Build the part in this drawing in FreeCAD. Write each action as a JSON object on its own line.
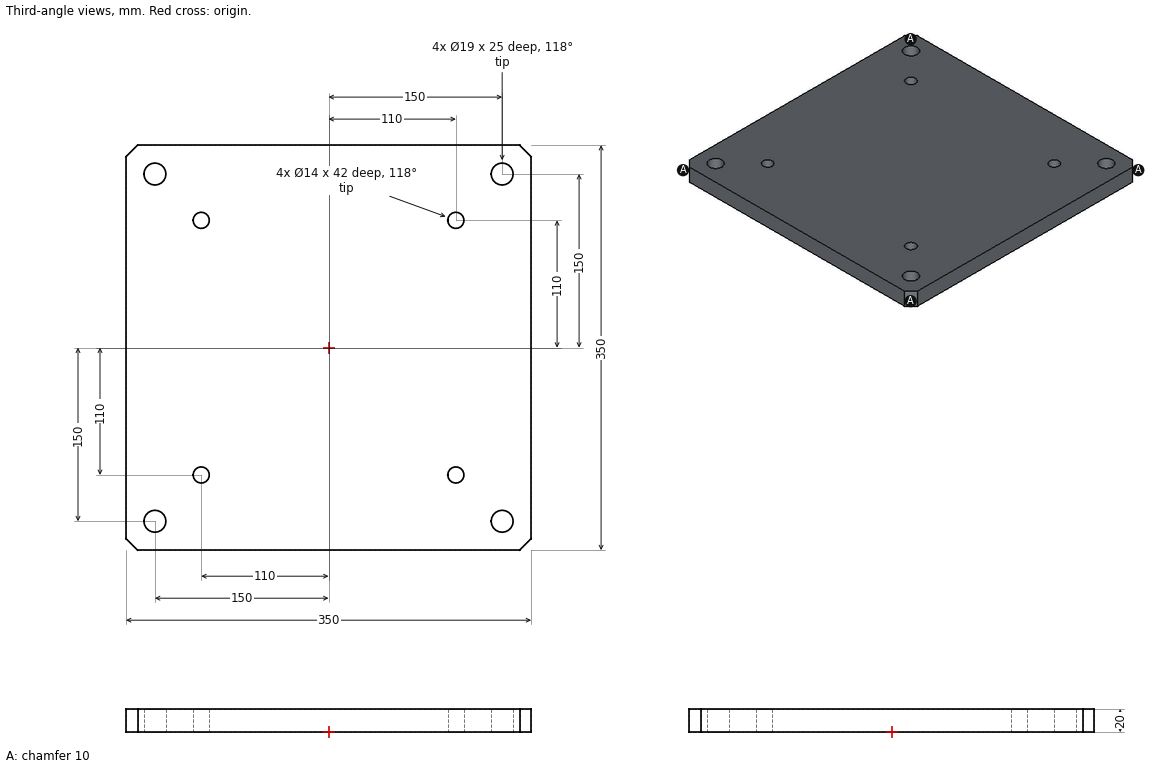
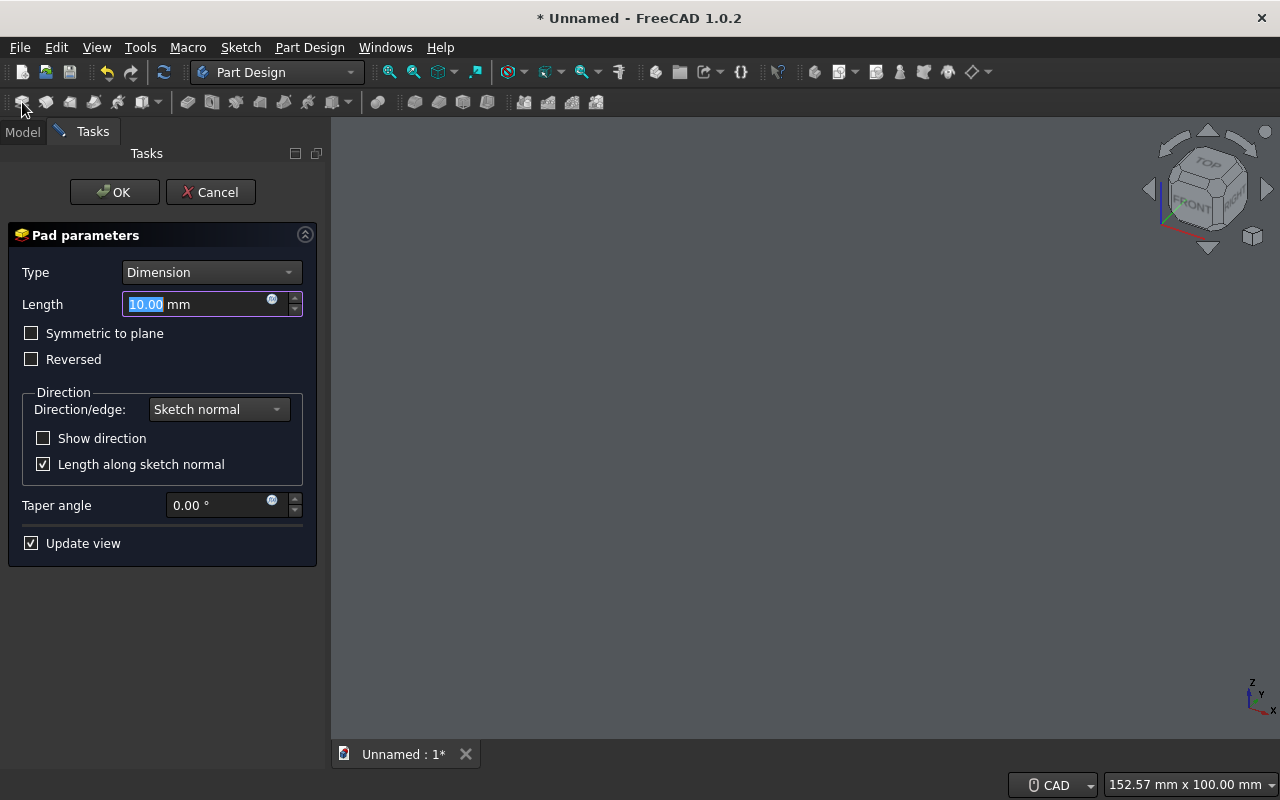
{"action": "type", "text": "20"}
{"action": "key", "text": "Tab"}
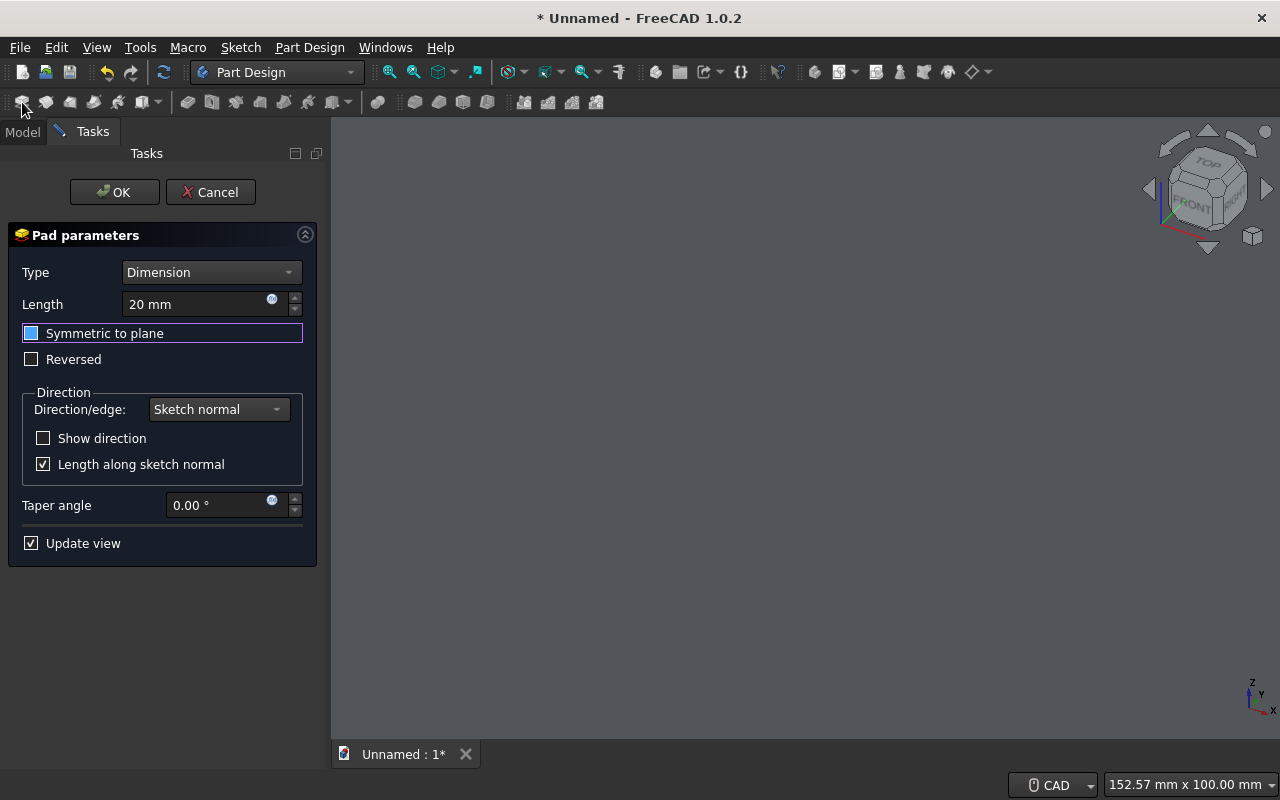
{"action": "left_click", "coordinate": [115, 192]}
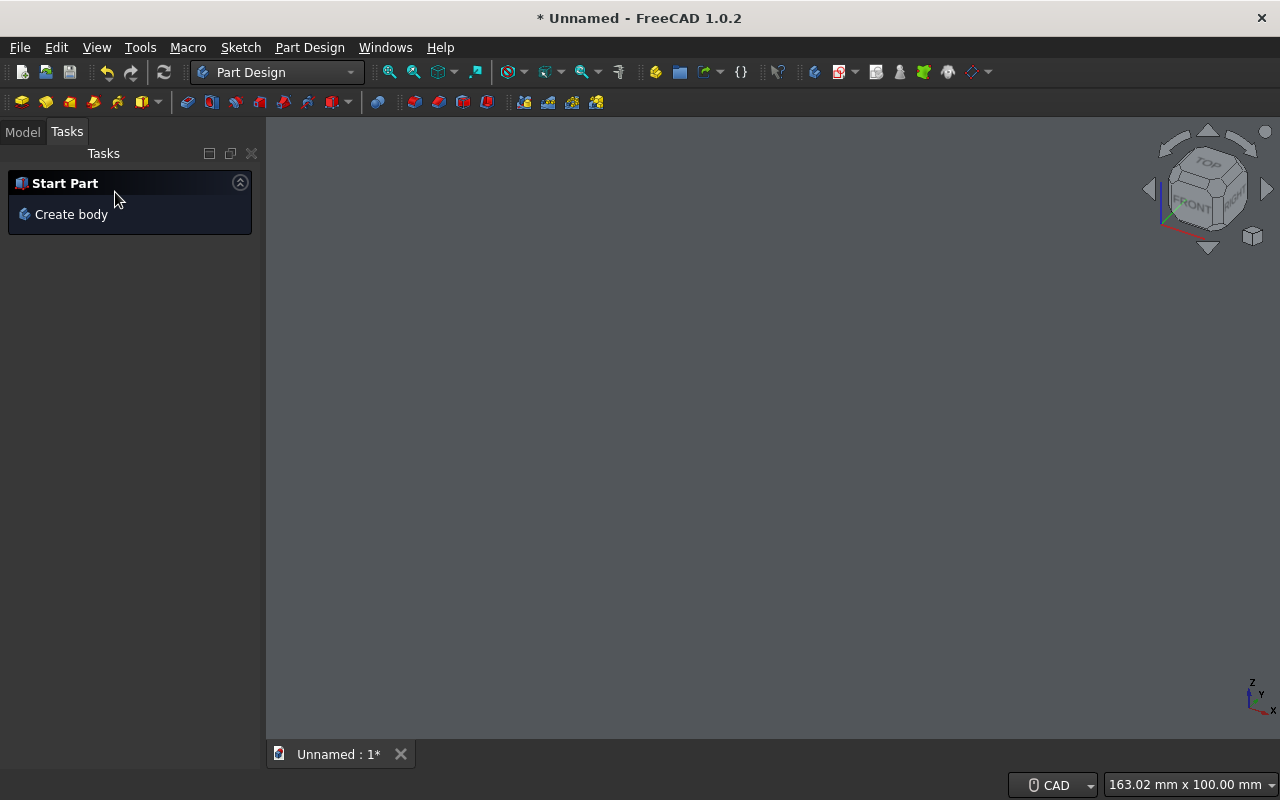
{"action": "left_click", "coordinate": [390, 72]}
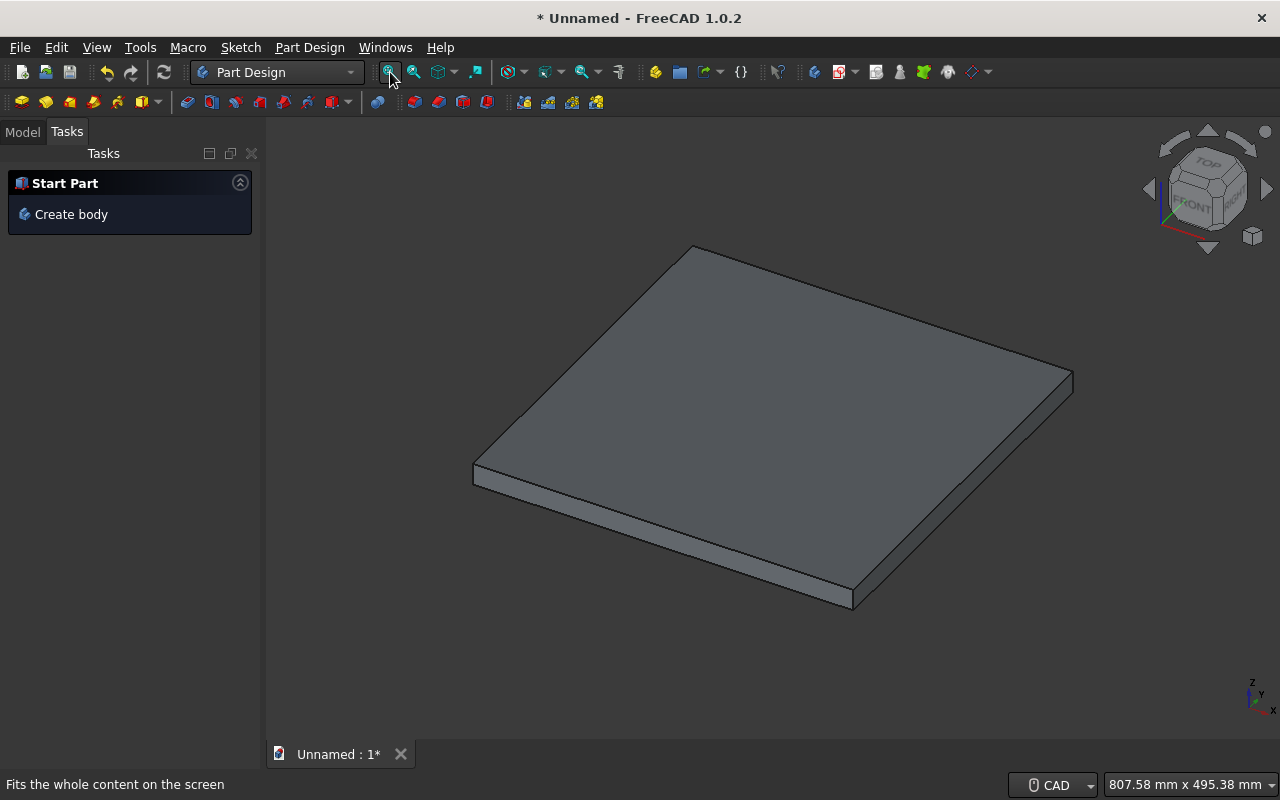
{"action": "left_click", "coordinate": [773, 417]}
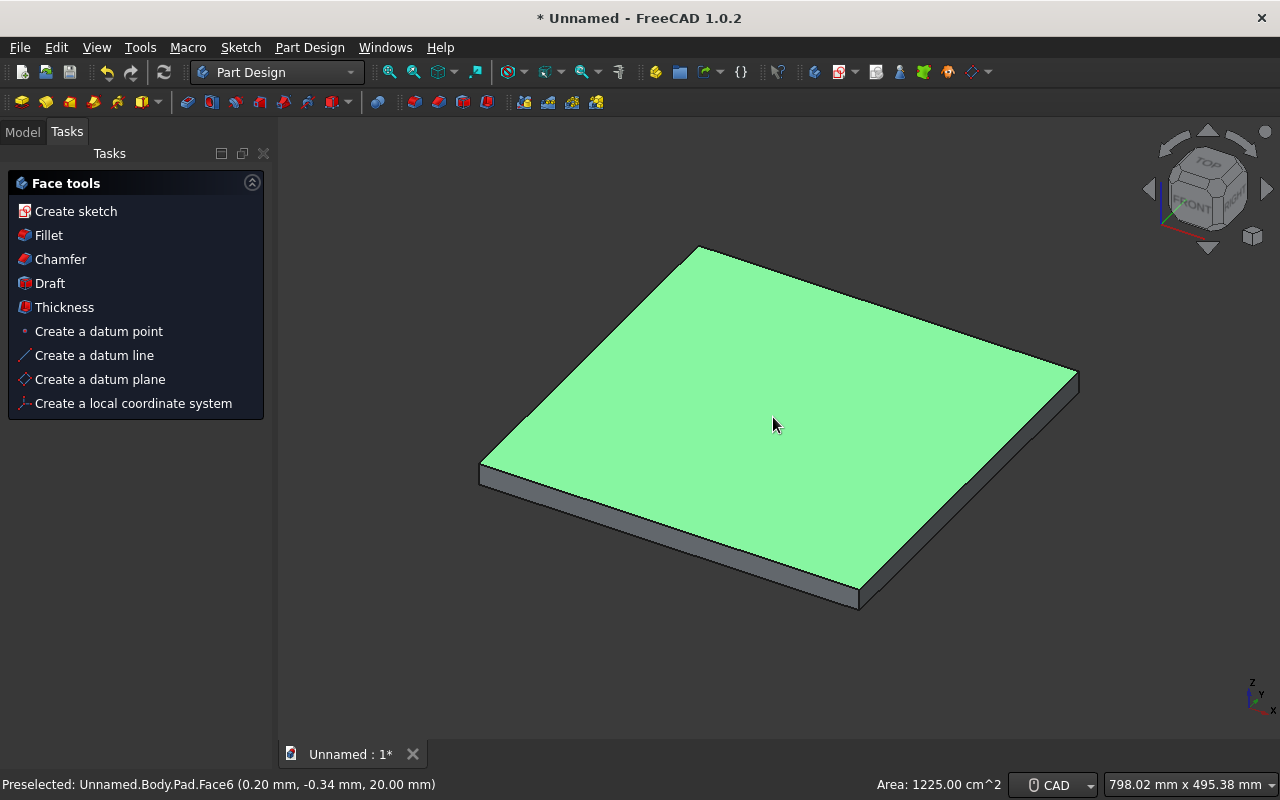
{"action": "left_click", "coordinate": [840, 72]}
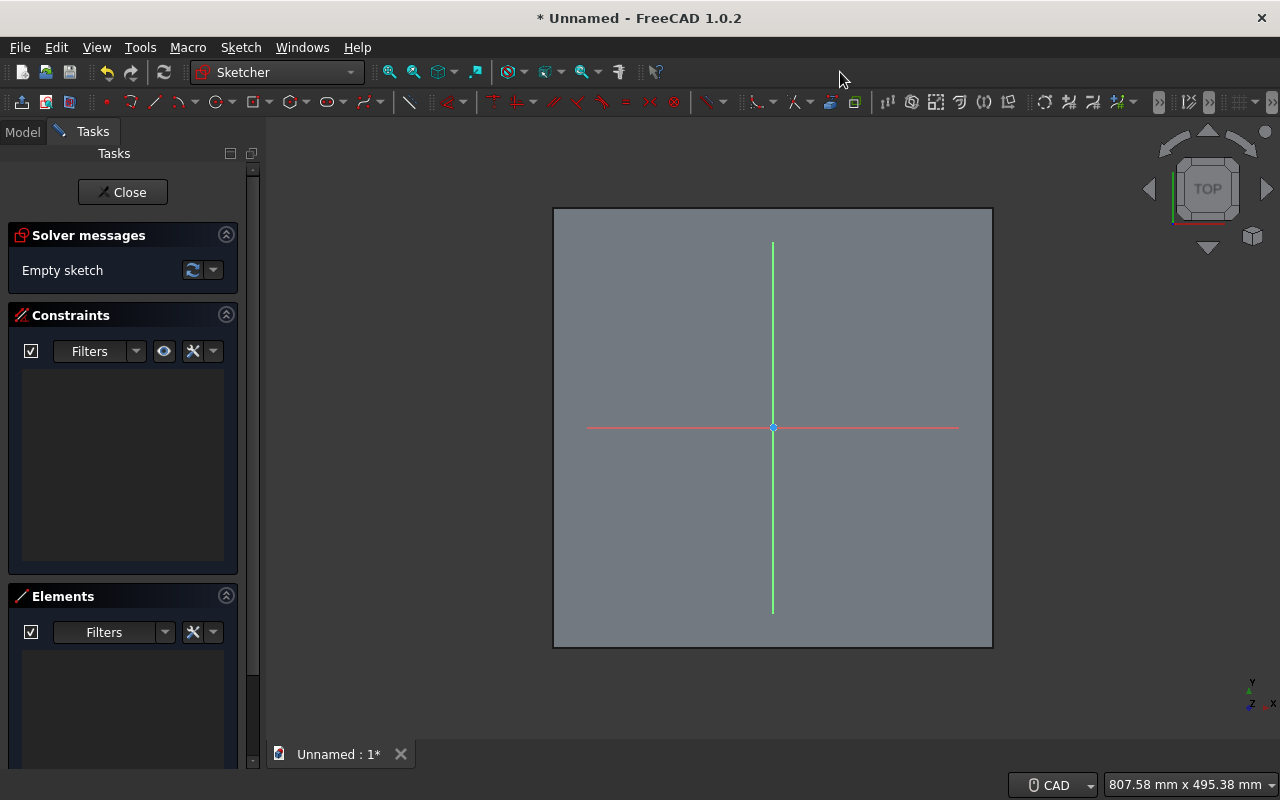
{"action": "scroll", "coordinate": [912, 428], "scroll_direction": "up", "scroll_amount": 2}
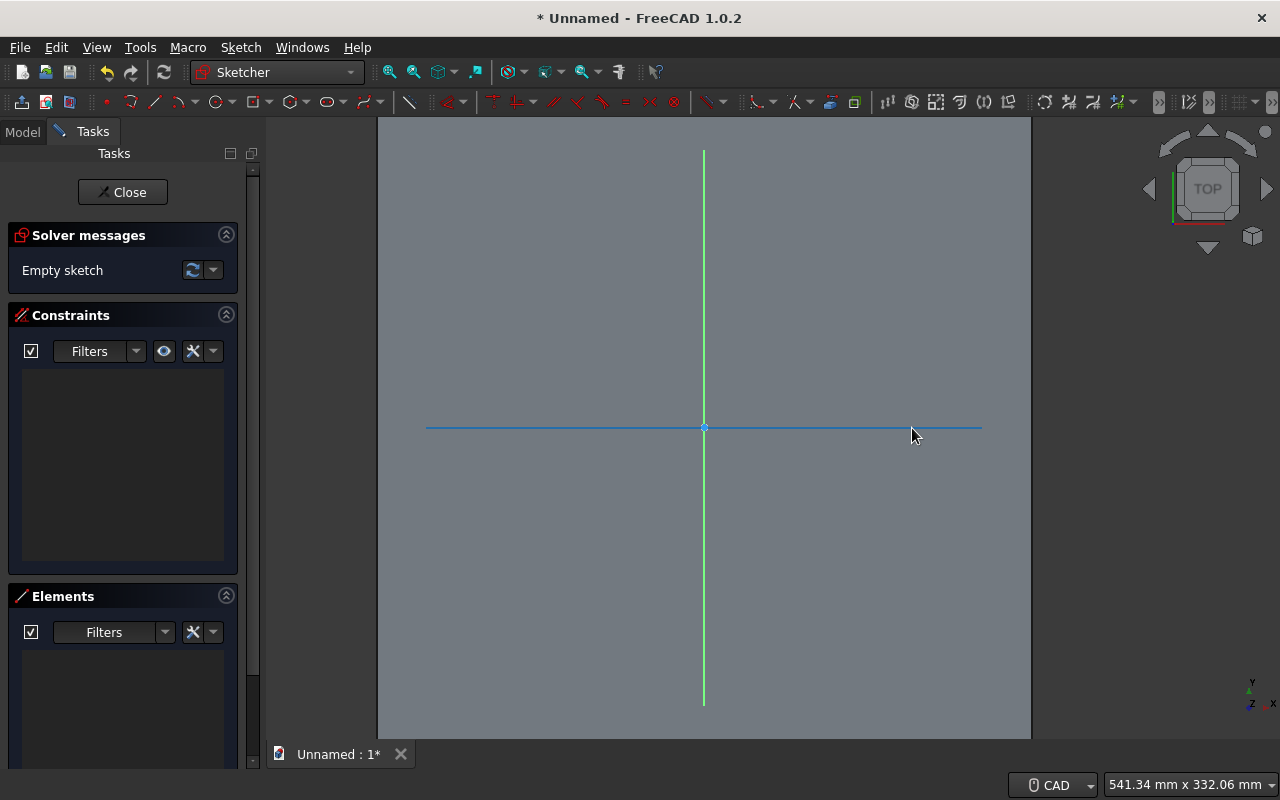
{"action": "key", "text": "g c"}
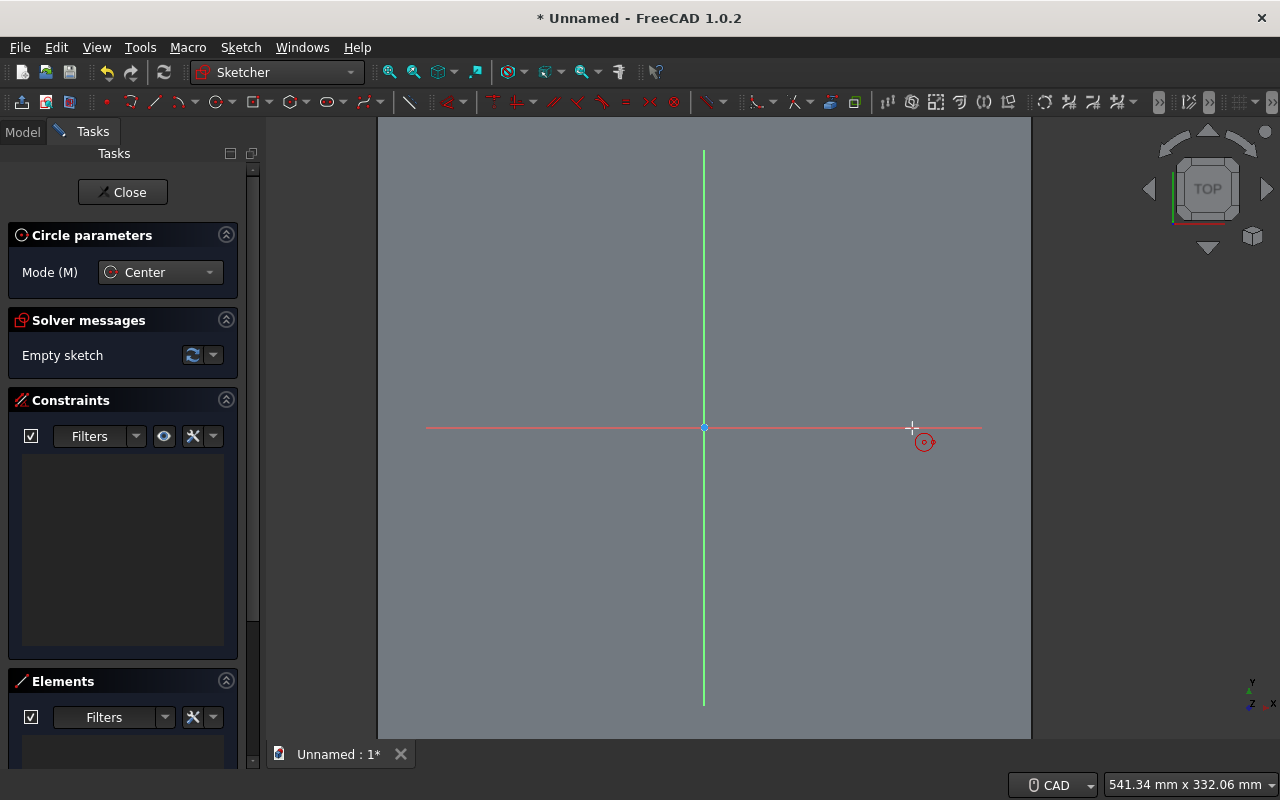
{"action": "scroll", "coordinate": [910, 222], "scroll_direction": "up", "scroll_amount": 3}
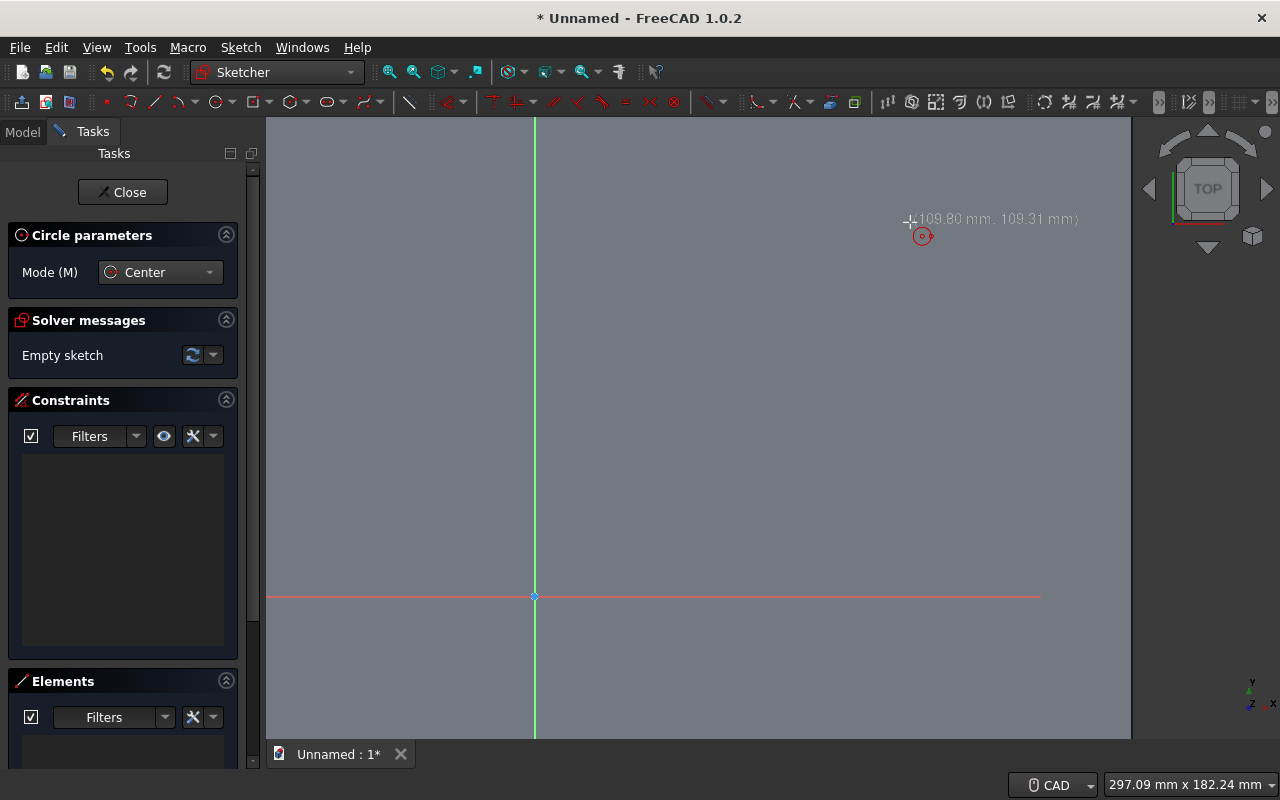
{"action": "left_click", "coordinate": [910, 221]}
{"action": "mouse_move", "coordinate": [927, 204]}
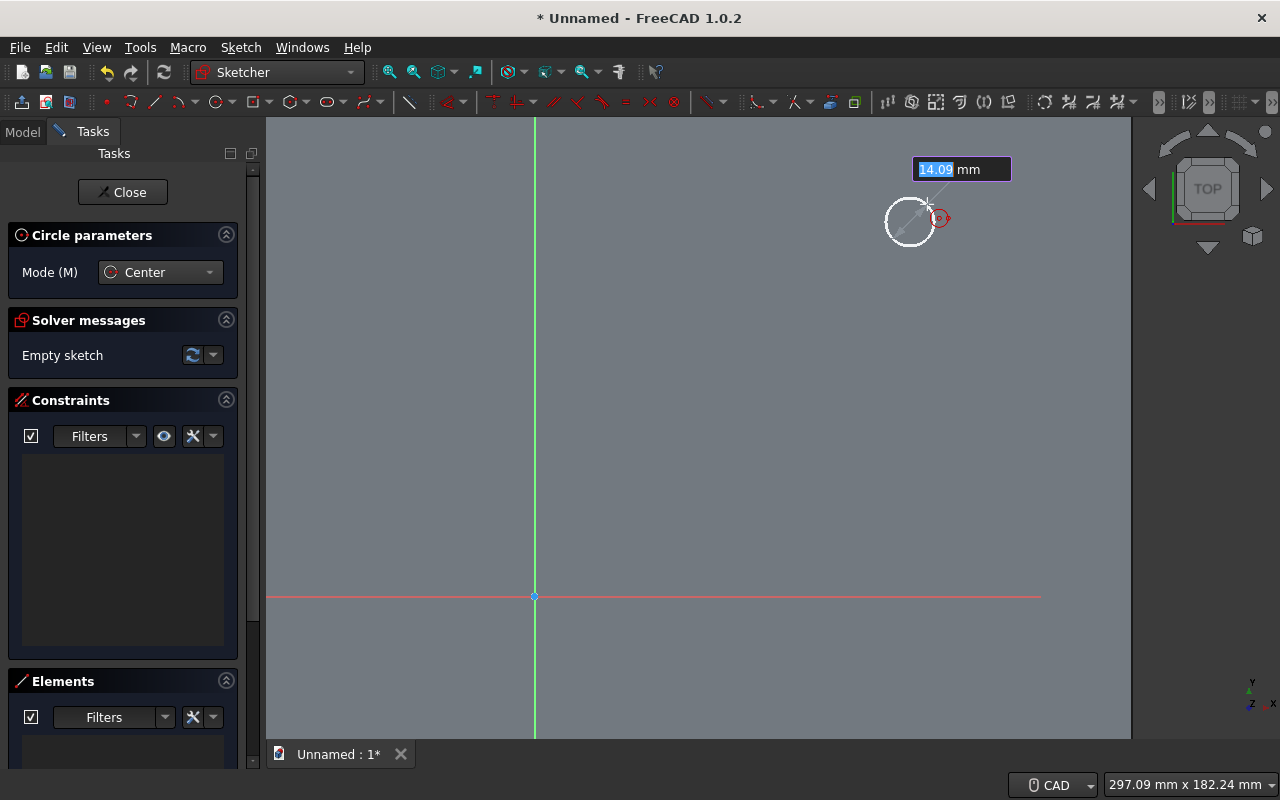
{"action": "type", "text": "14"}
{"action": "key", "text": "Return"}